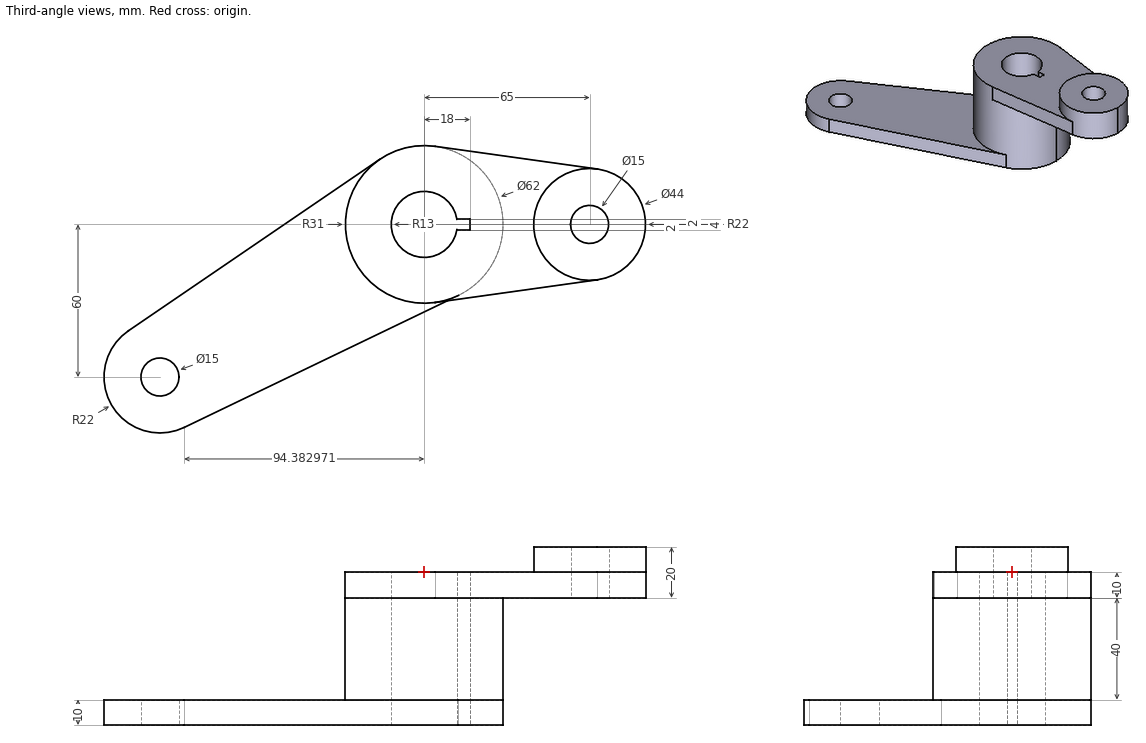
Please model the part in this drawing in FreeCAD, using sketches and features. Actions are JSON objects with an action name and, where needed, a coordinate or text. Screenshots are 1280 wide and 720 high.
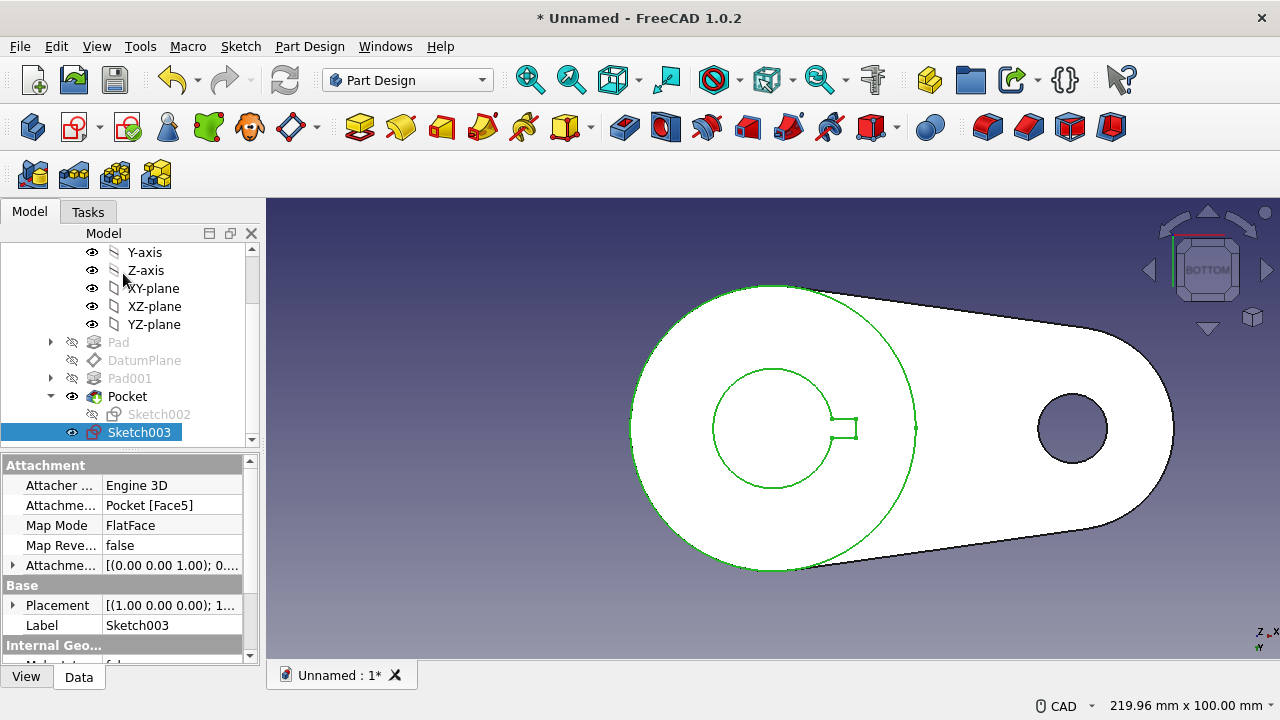
{"action": "left_click", "coordinate": [360, 128]}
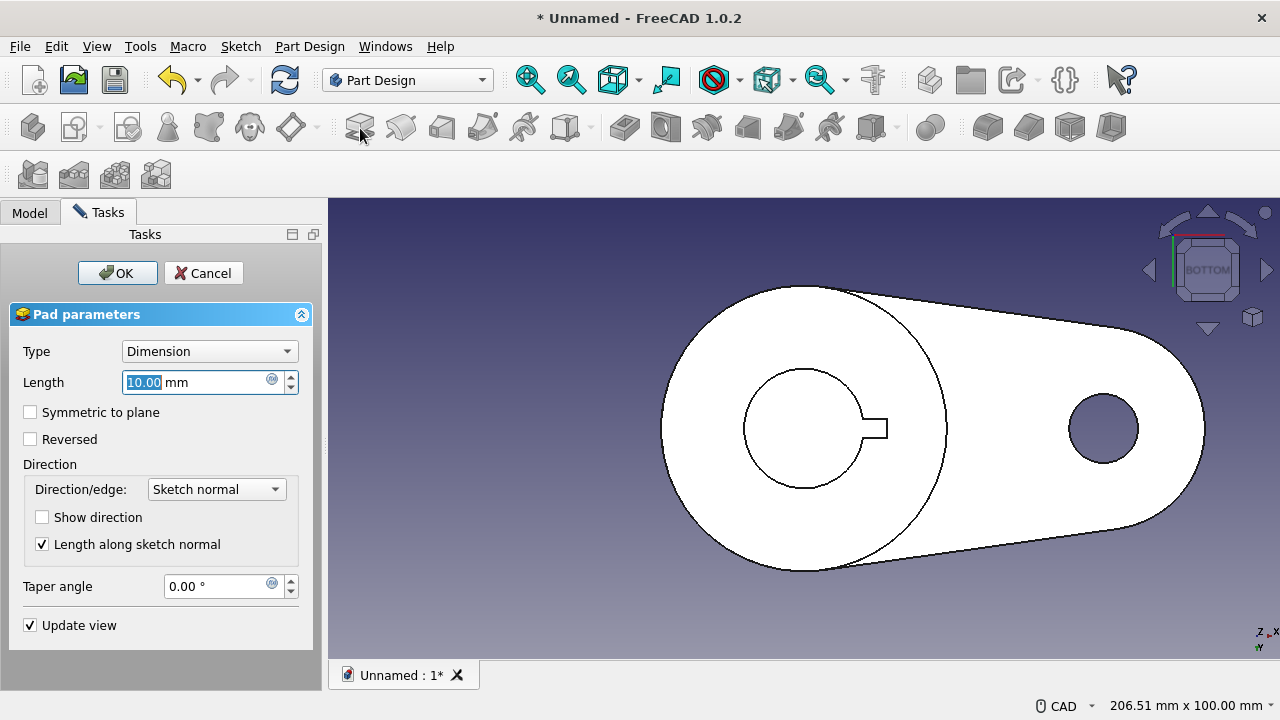
{"action": "type", "text": "40"}
{"action": "key", "text": "Tab"}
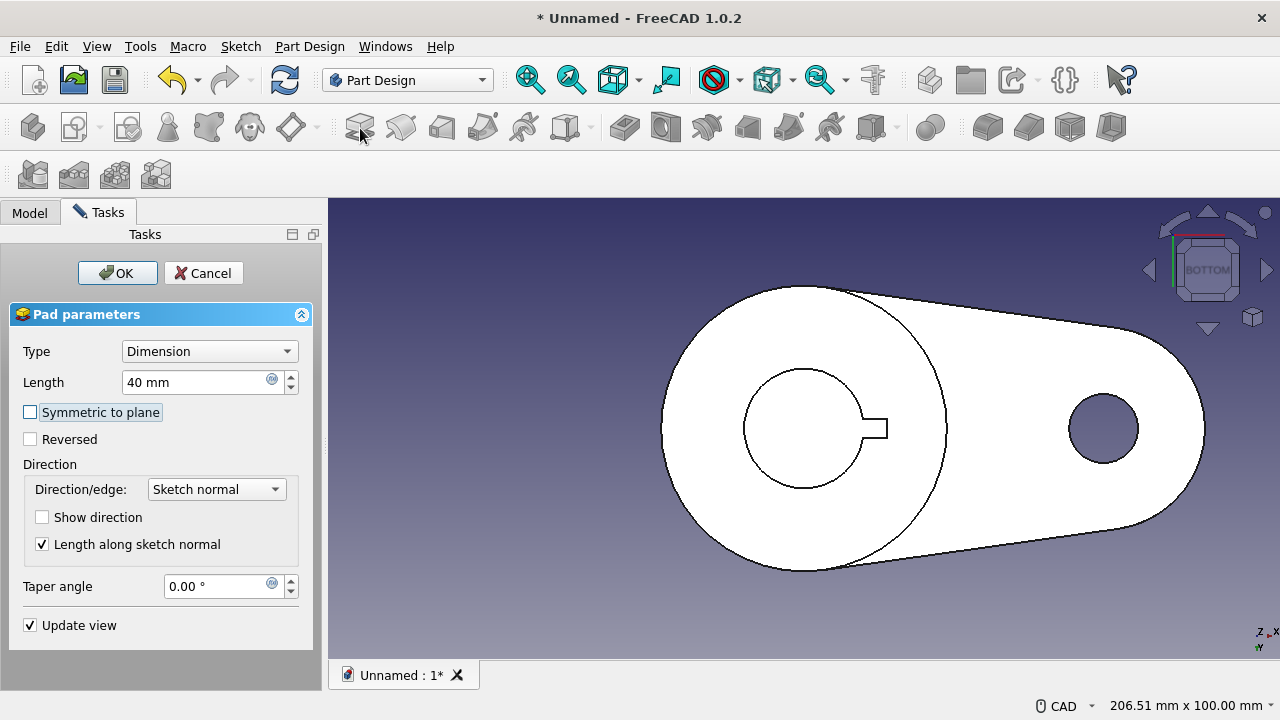
{"action": "left_click", "coordinate": [118, 273]}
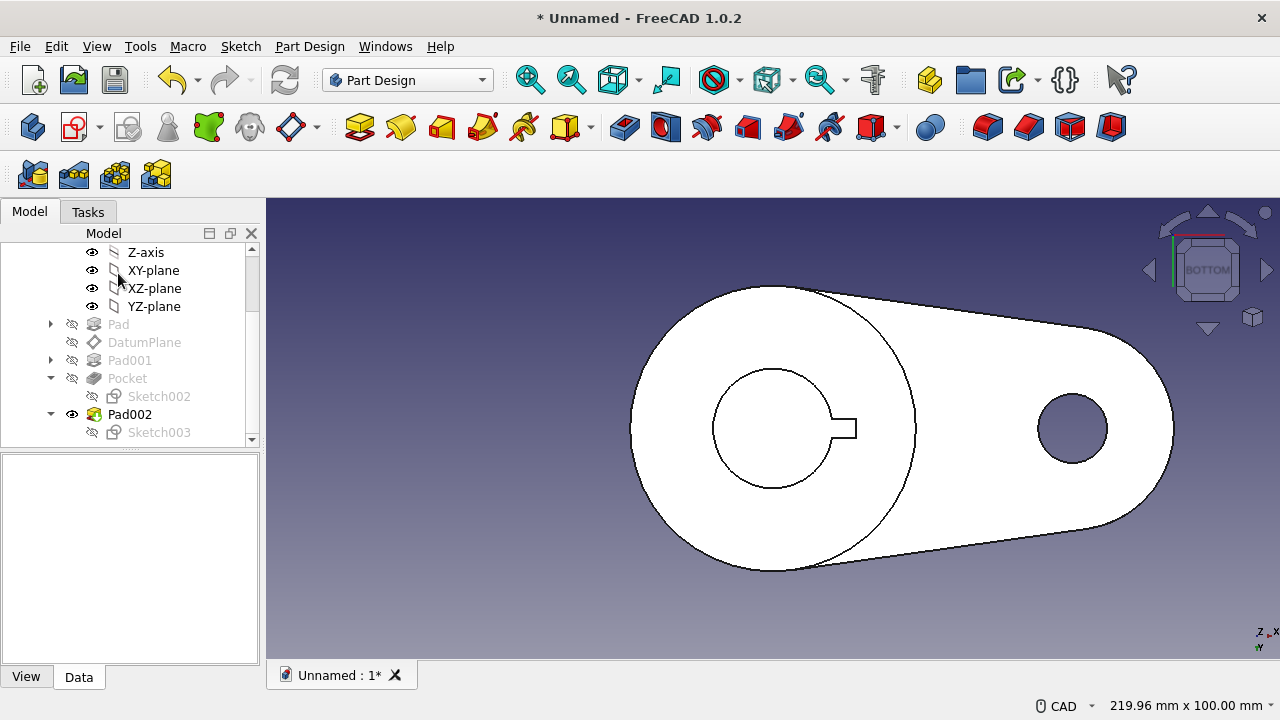
{"action": "left_click", "coordinate": [983, 468]}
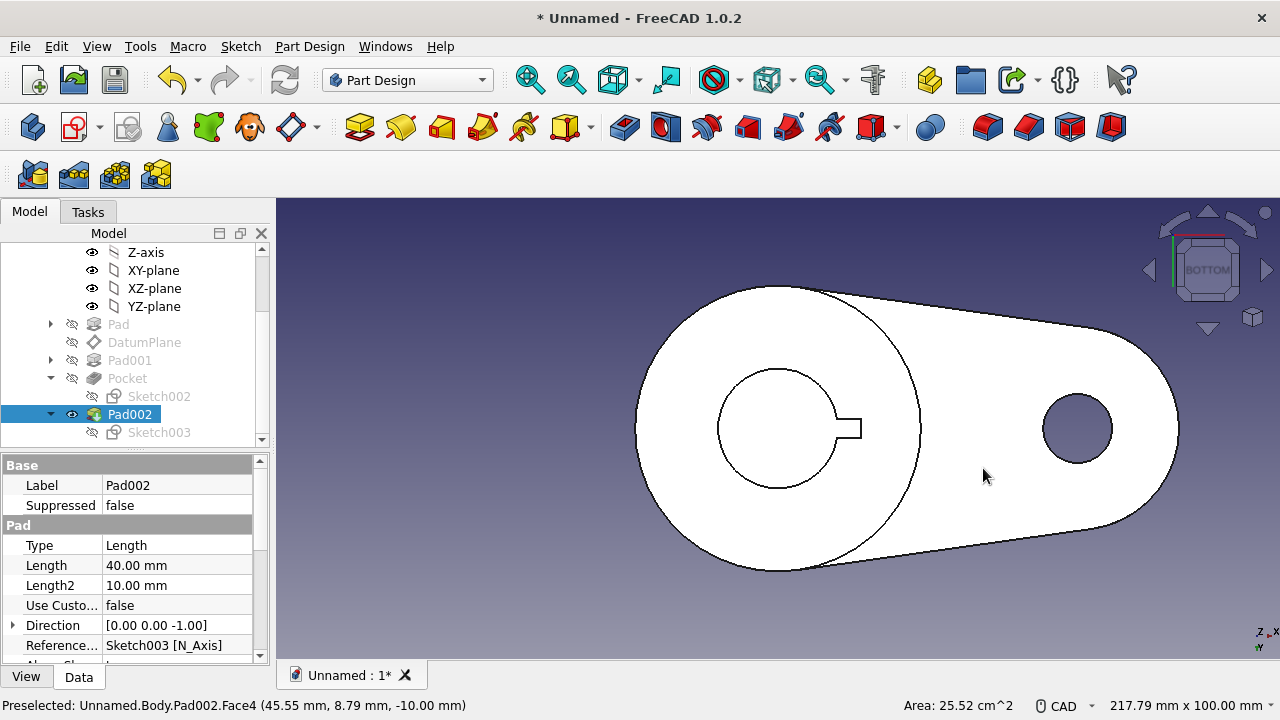
{"action": "left_click", "coordinate": [74, 128]}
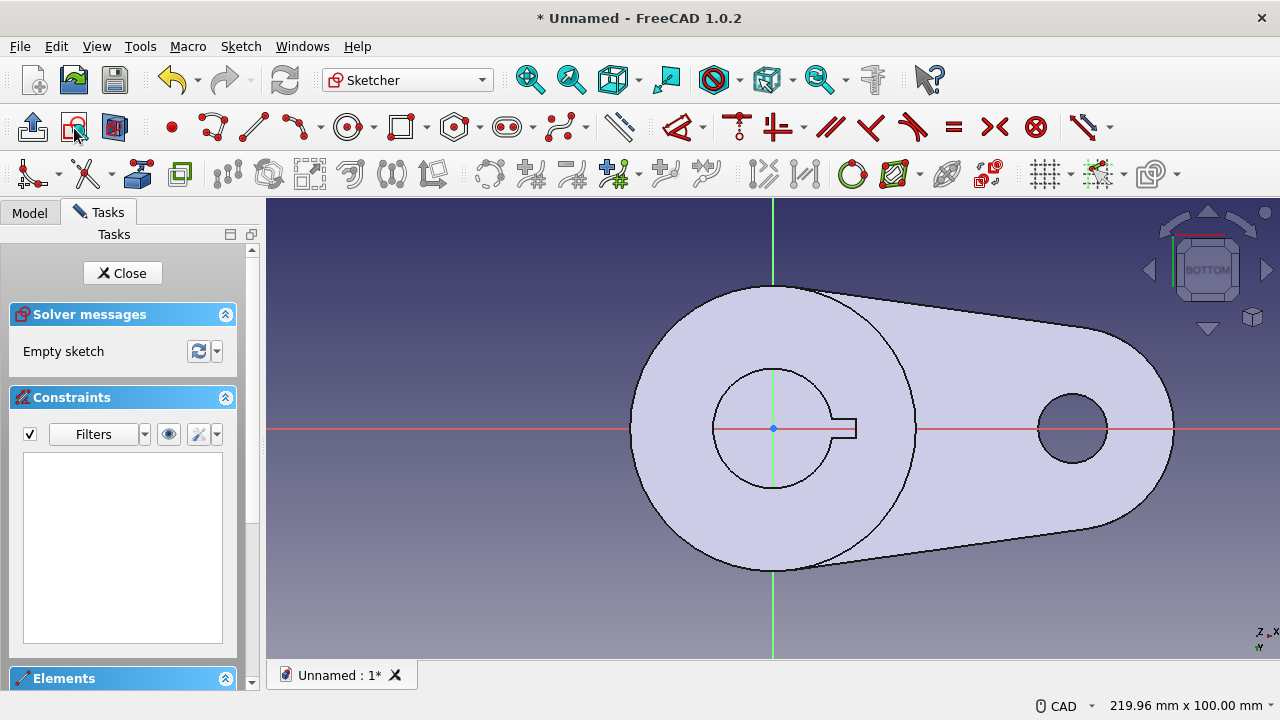
{"action": "key", "text": "q s"}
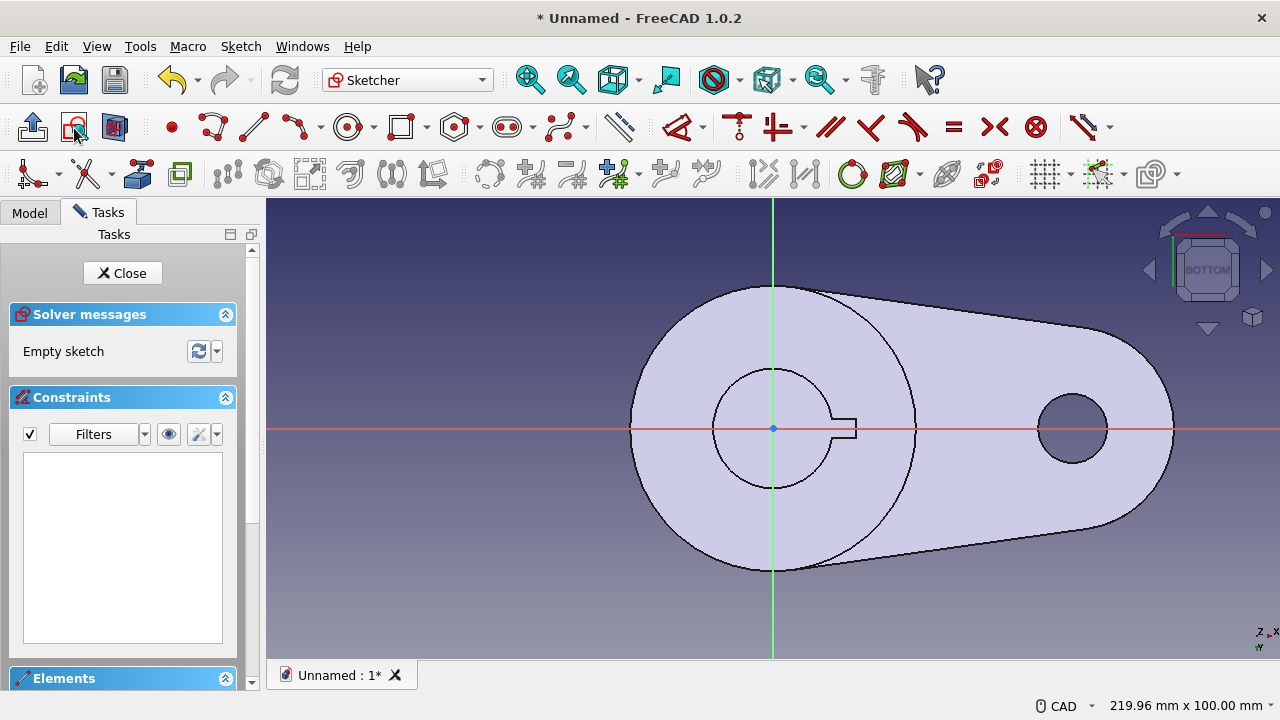
{"action": "scroll", "coordinate": [811, 429], "scroll_direction": "up", "scroll_amount": 7}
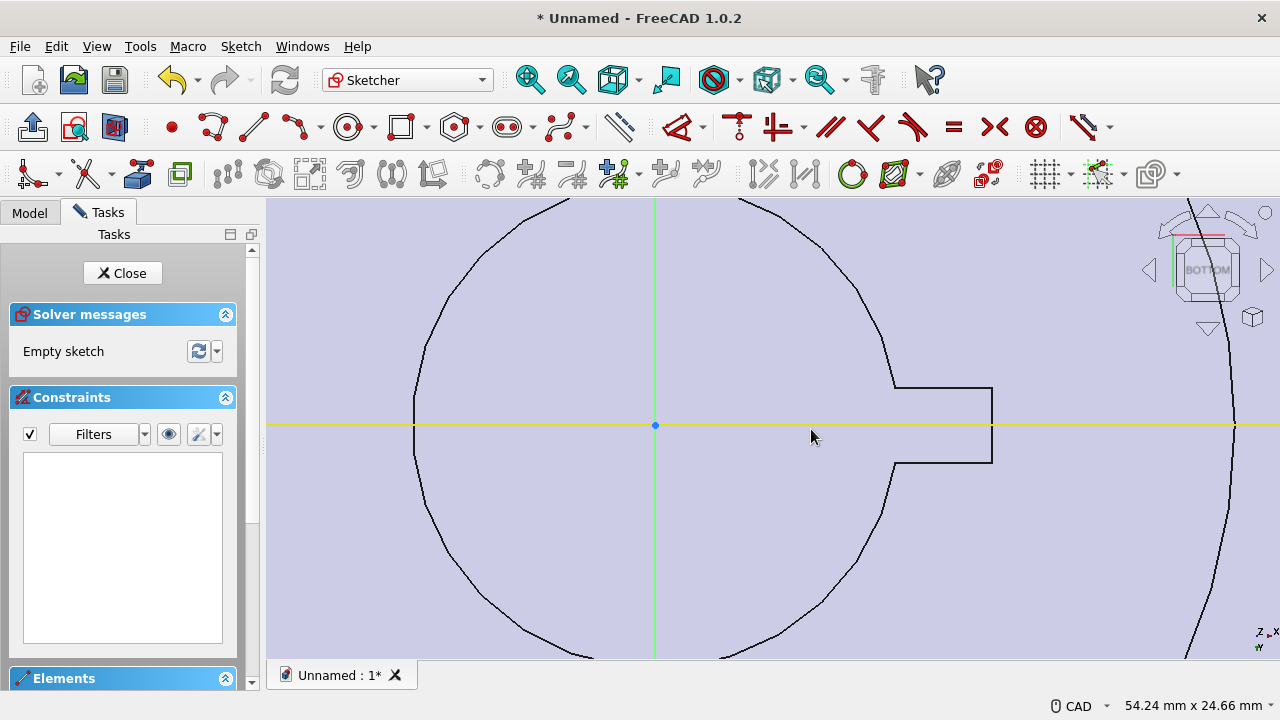
{"action": "left_click", "coordinate": [213, 128]}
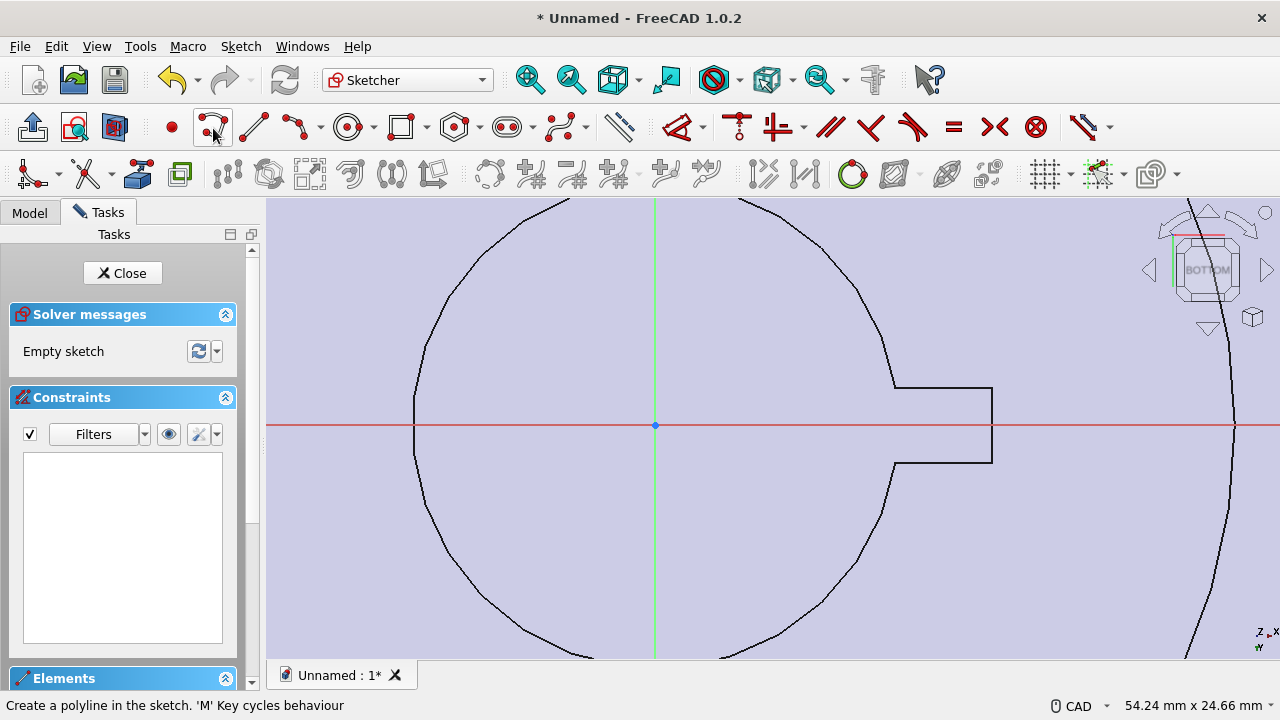
{"action": "left_click", "coordinate": [895, 463]}
{"action": "left_click", "coordinate": [992, 463]}
{"action": "left_click", "coordinate": [992, 388]}
{"action": "left_click", "coordinate": [895, 388]}
{"action": "right_click", "coordinate": [895, 388]}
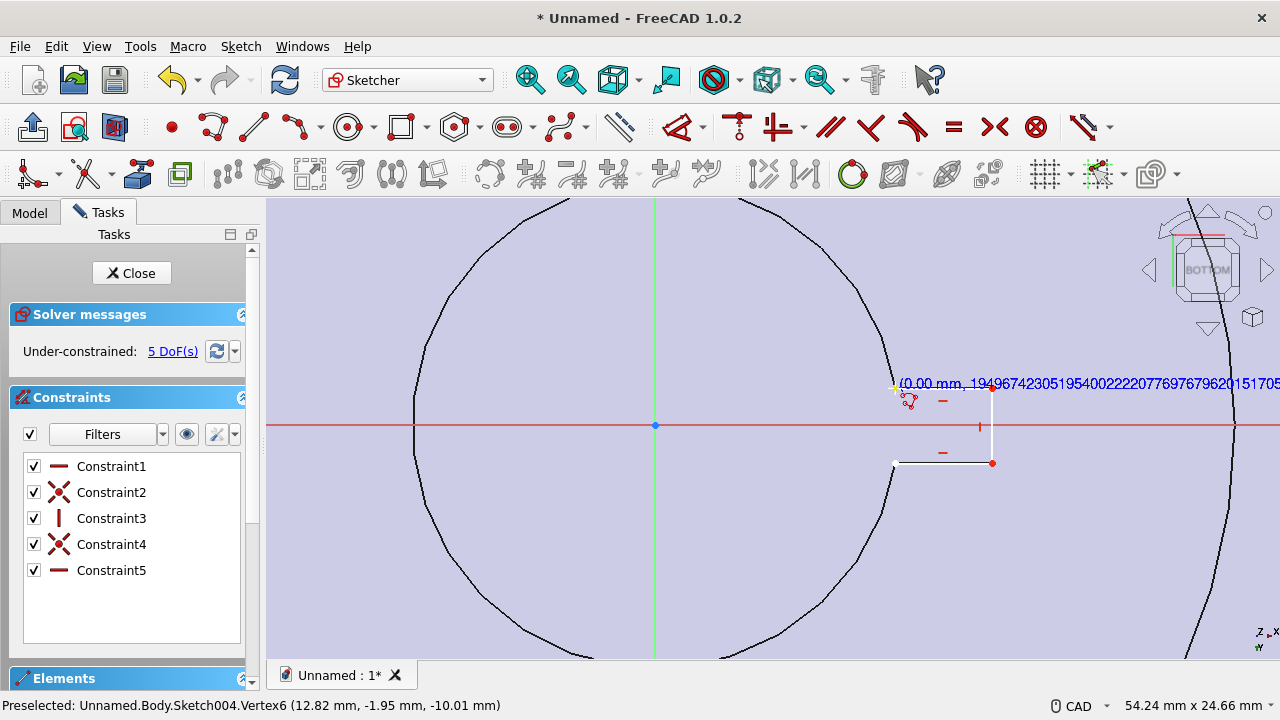
{"action": "key", "text": "g 3 a"}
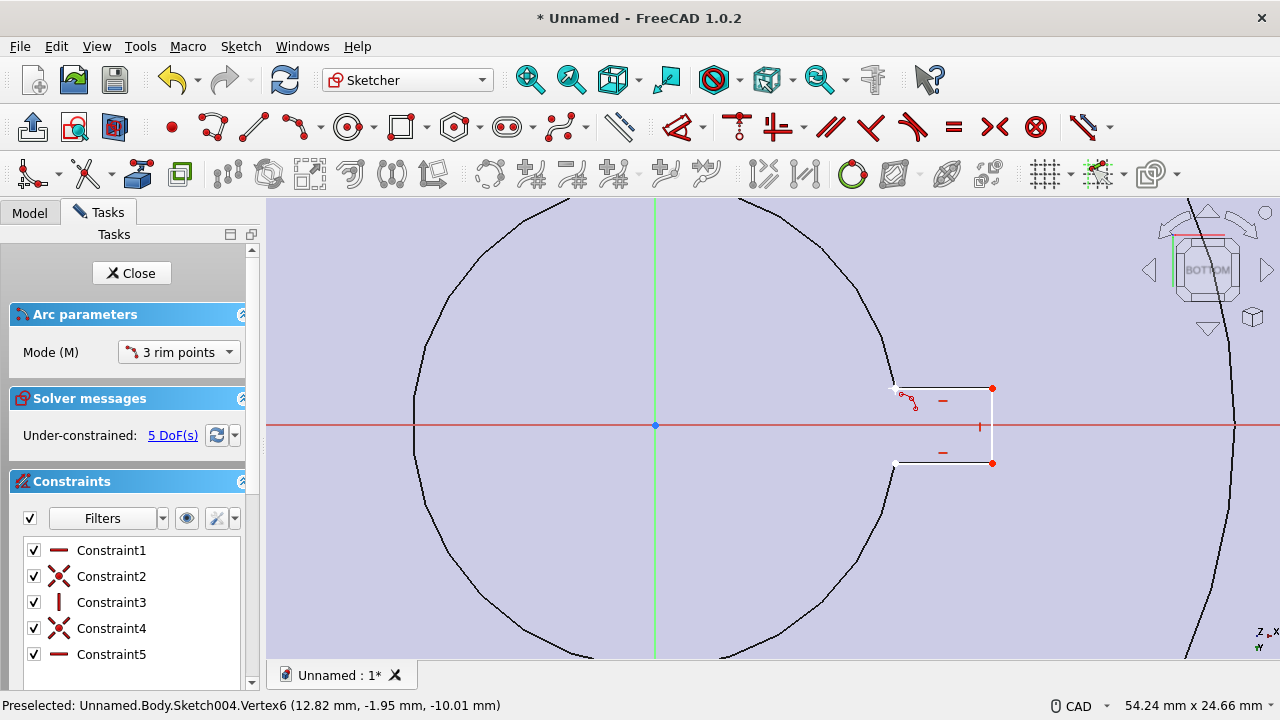
{"action": "left_click", "coordinate": [895, 389]}
{"action": "left_click", "coordinate": [895, 464]}
{"action": "left_click", "coordinate": [454, 289]}
{"action": "key", "text": "Escape"}